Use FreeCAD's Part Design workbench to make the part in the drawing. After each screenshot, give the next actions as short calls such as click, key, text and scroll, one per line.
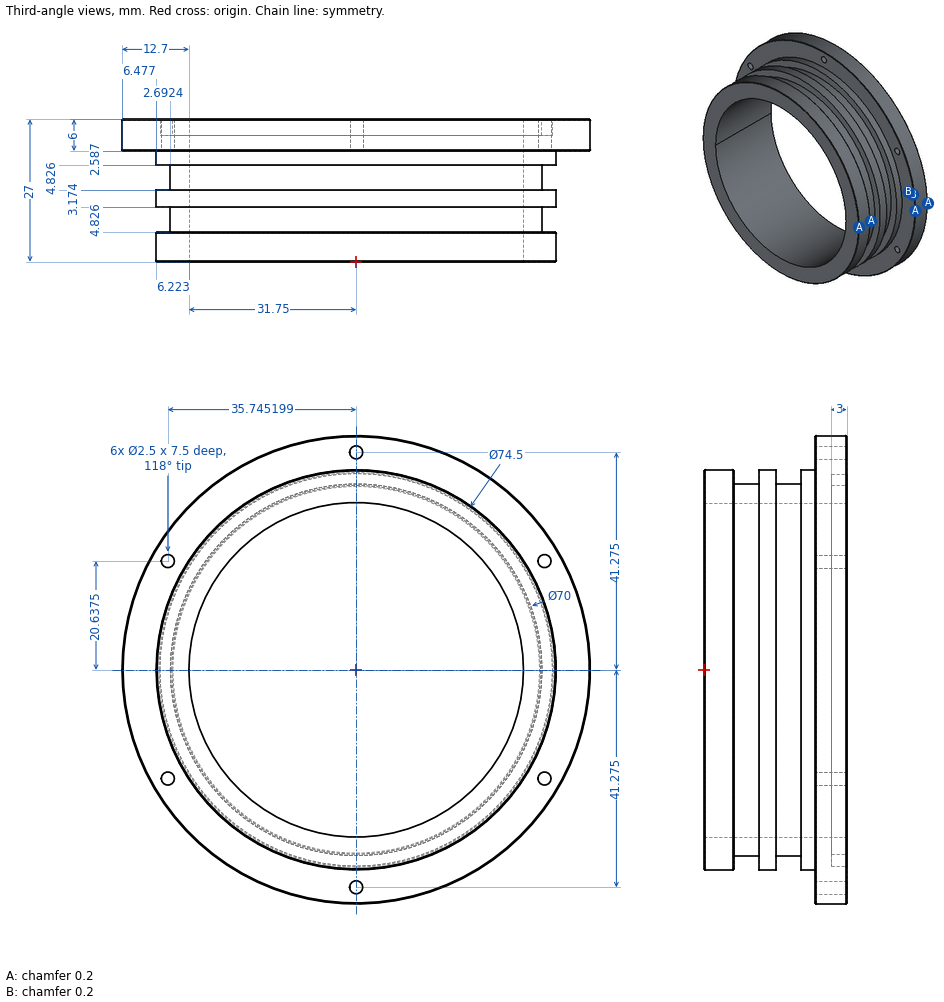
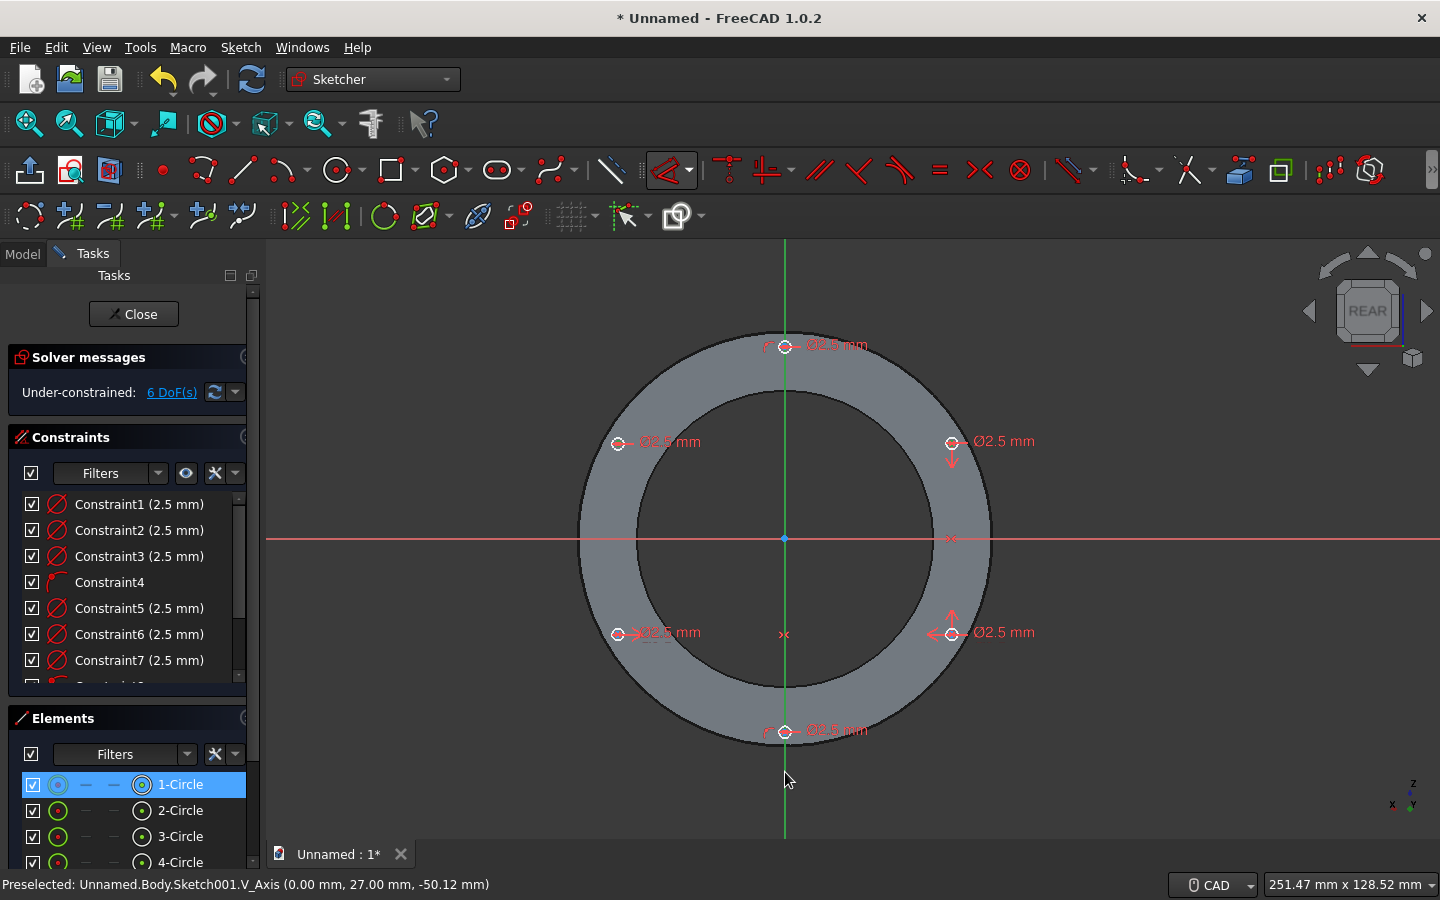
click(980, 170)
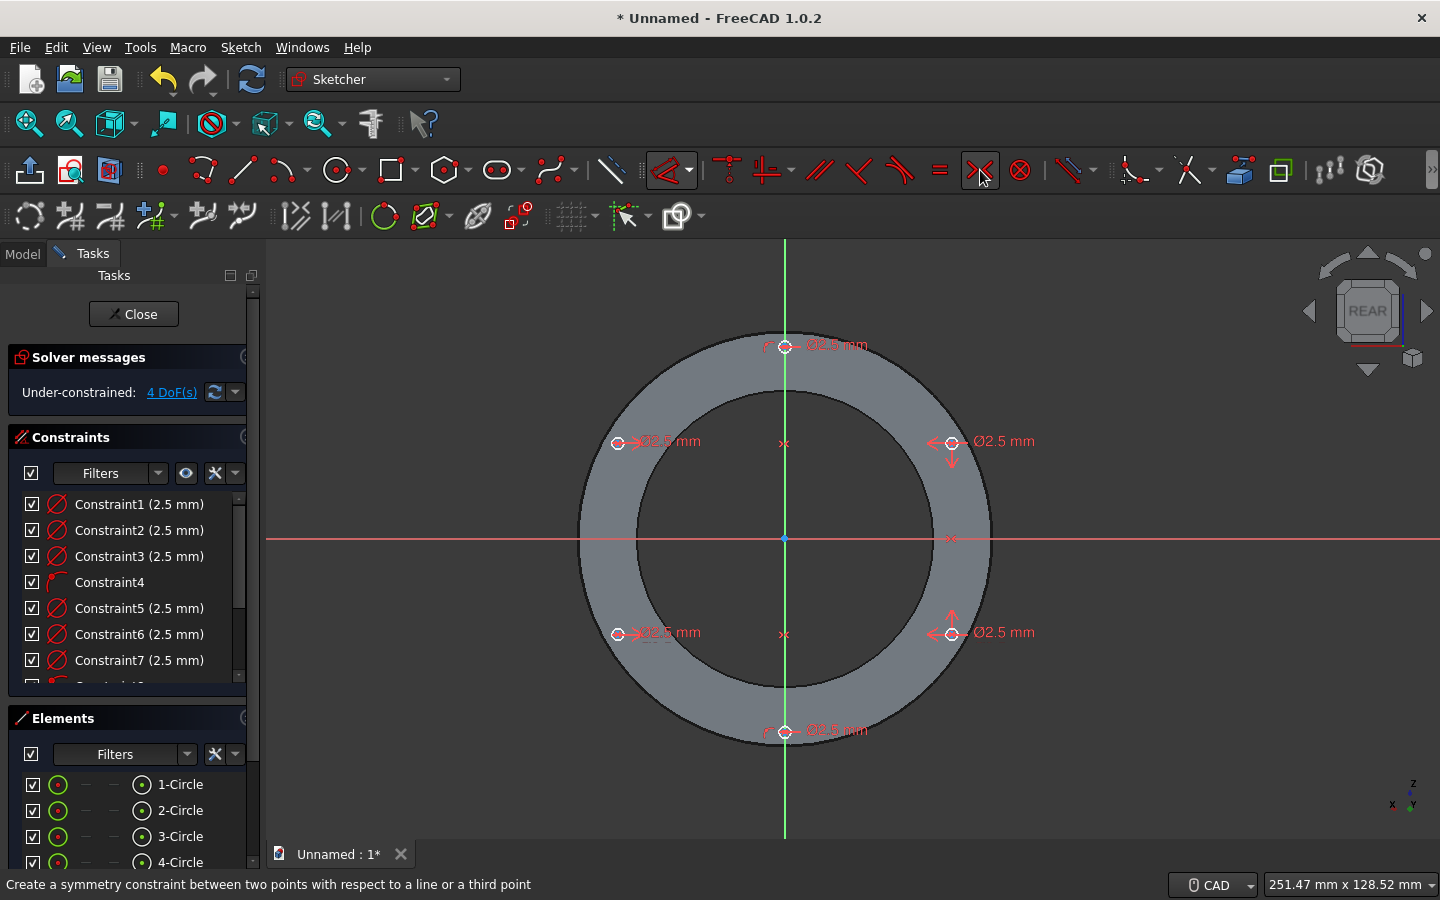
click(785, 732)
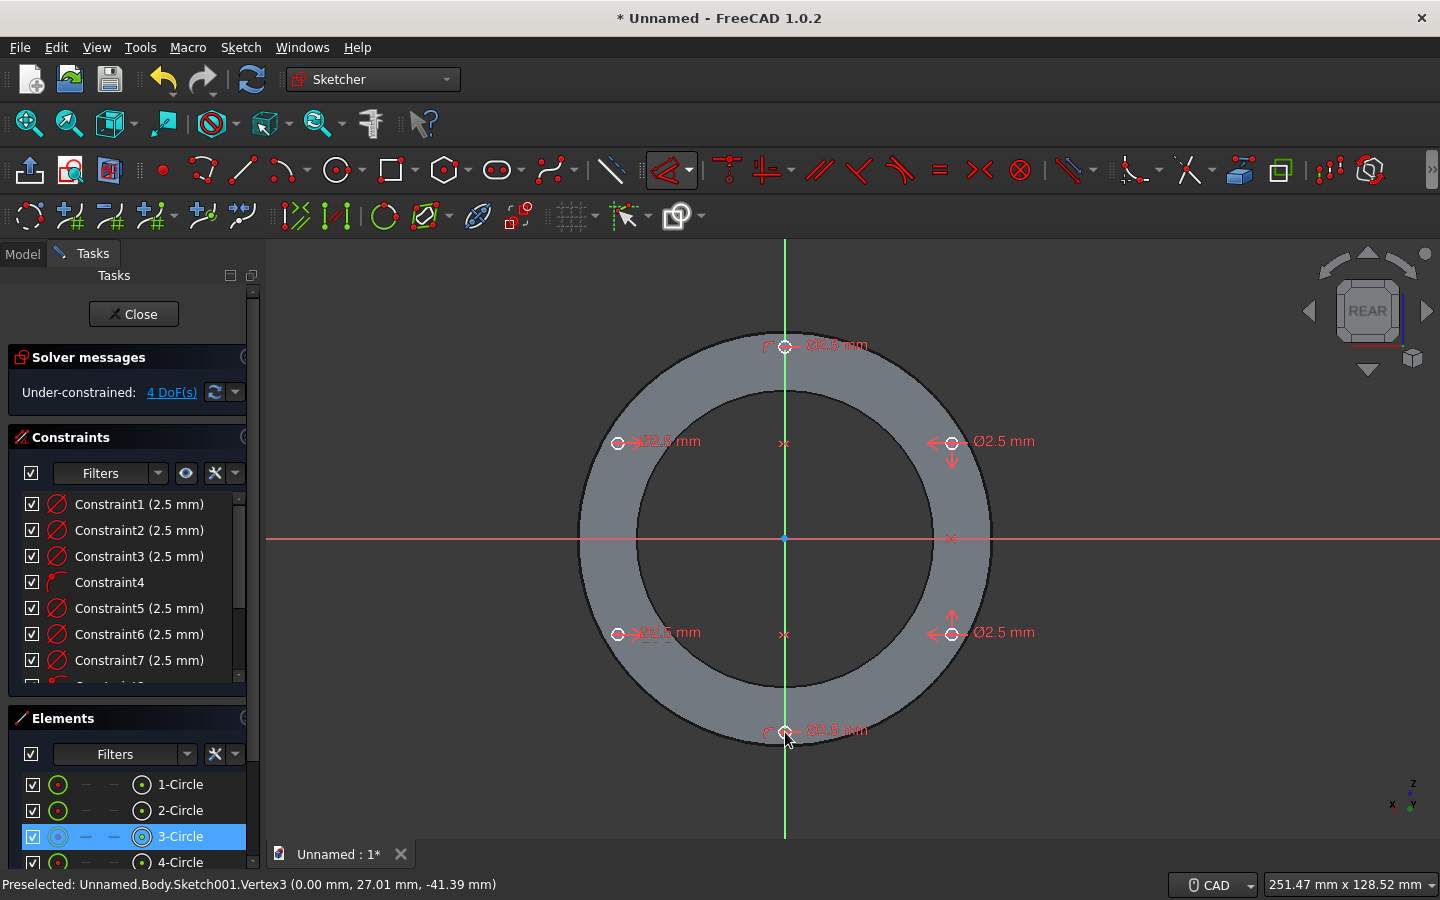
key(i)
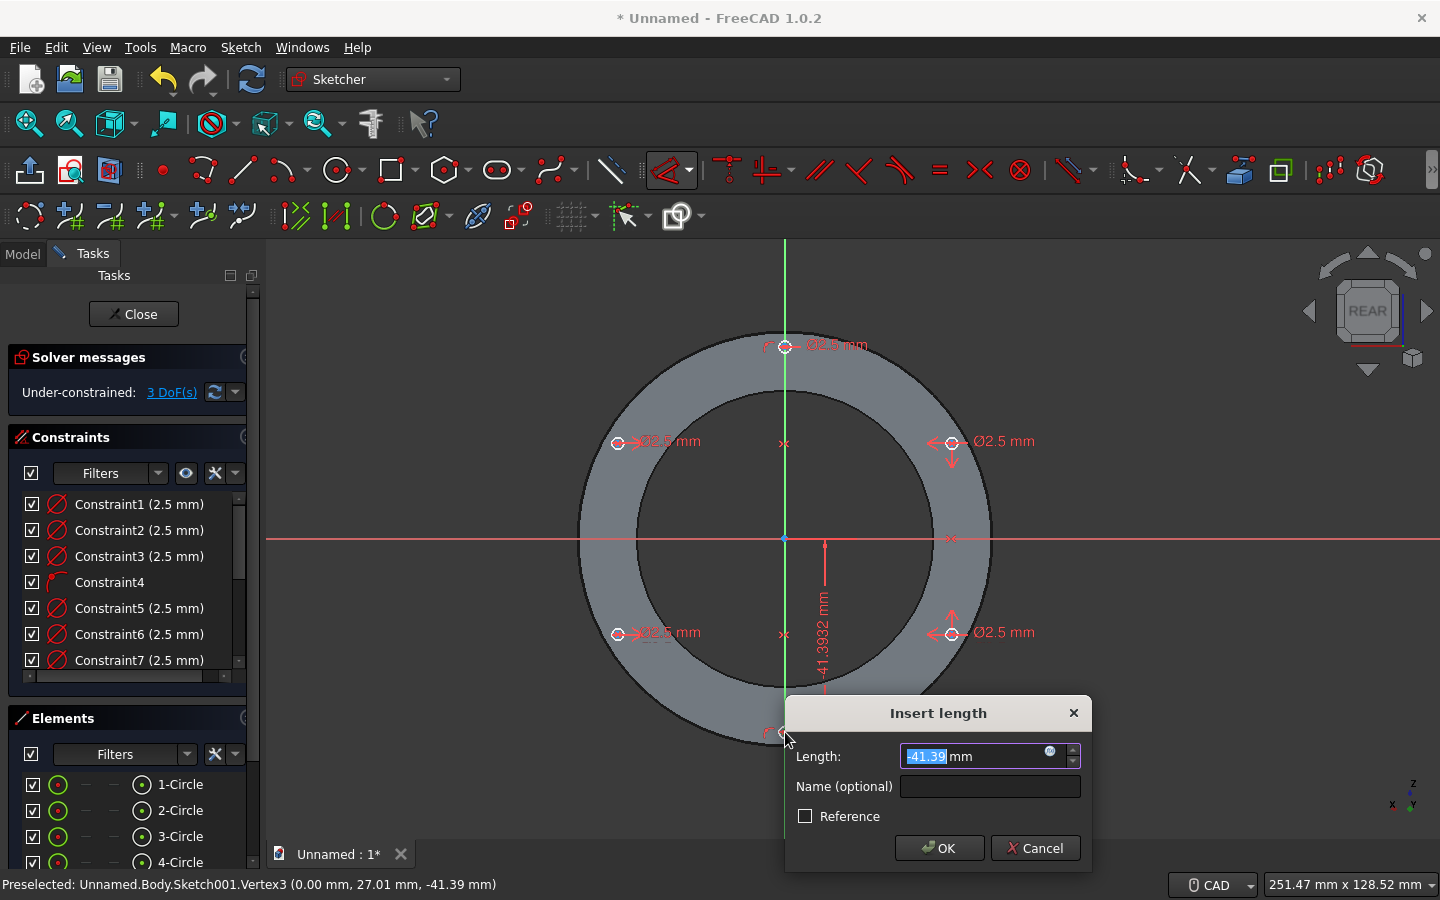
text(-41.275)
key(Return)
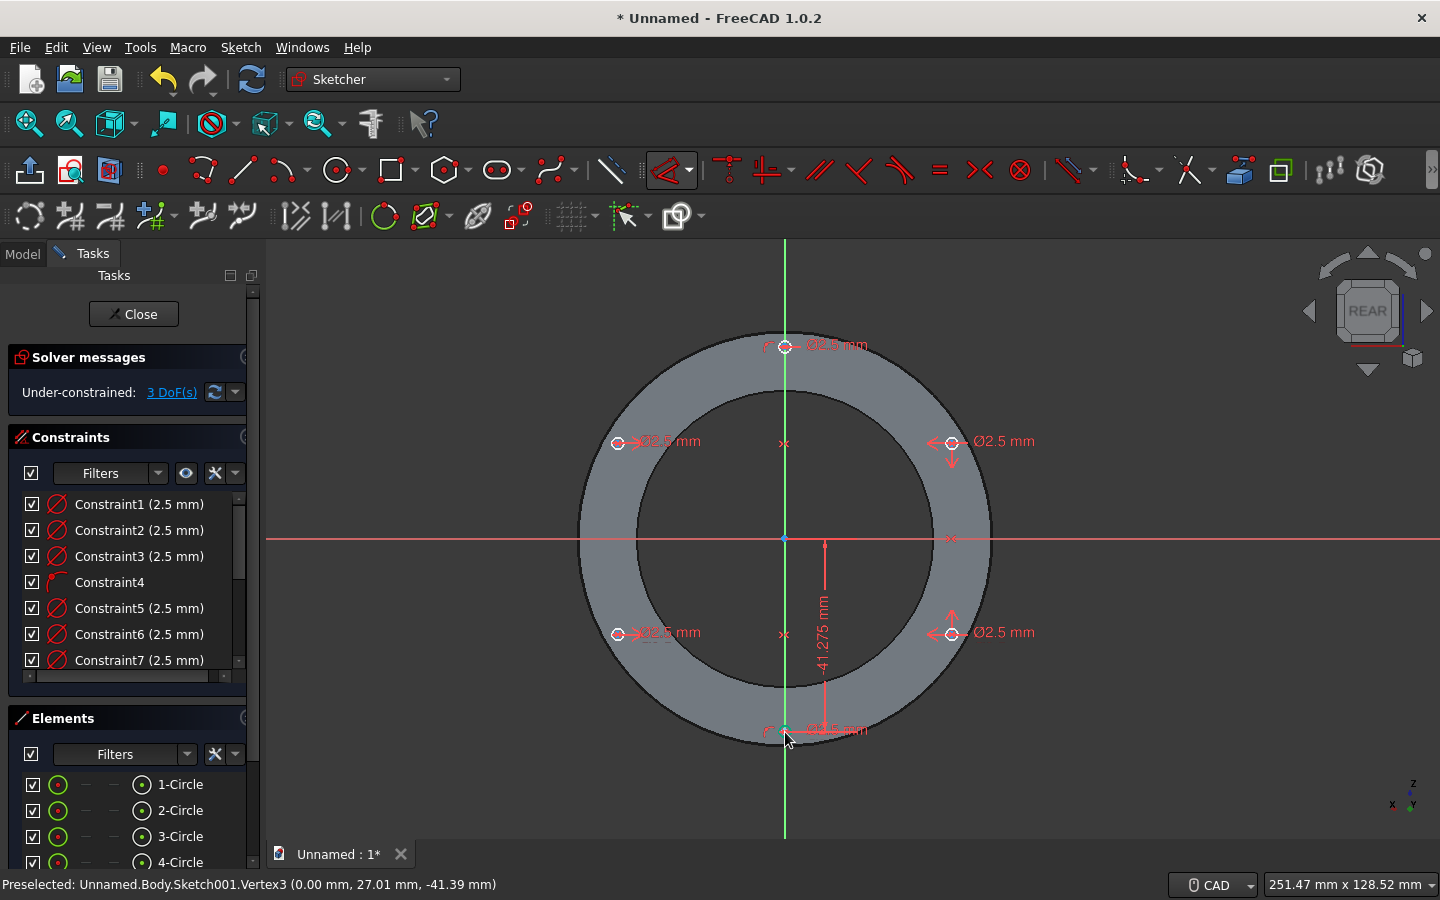
click(785, 347)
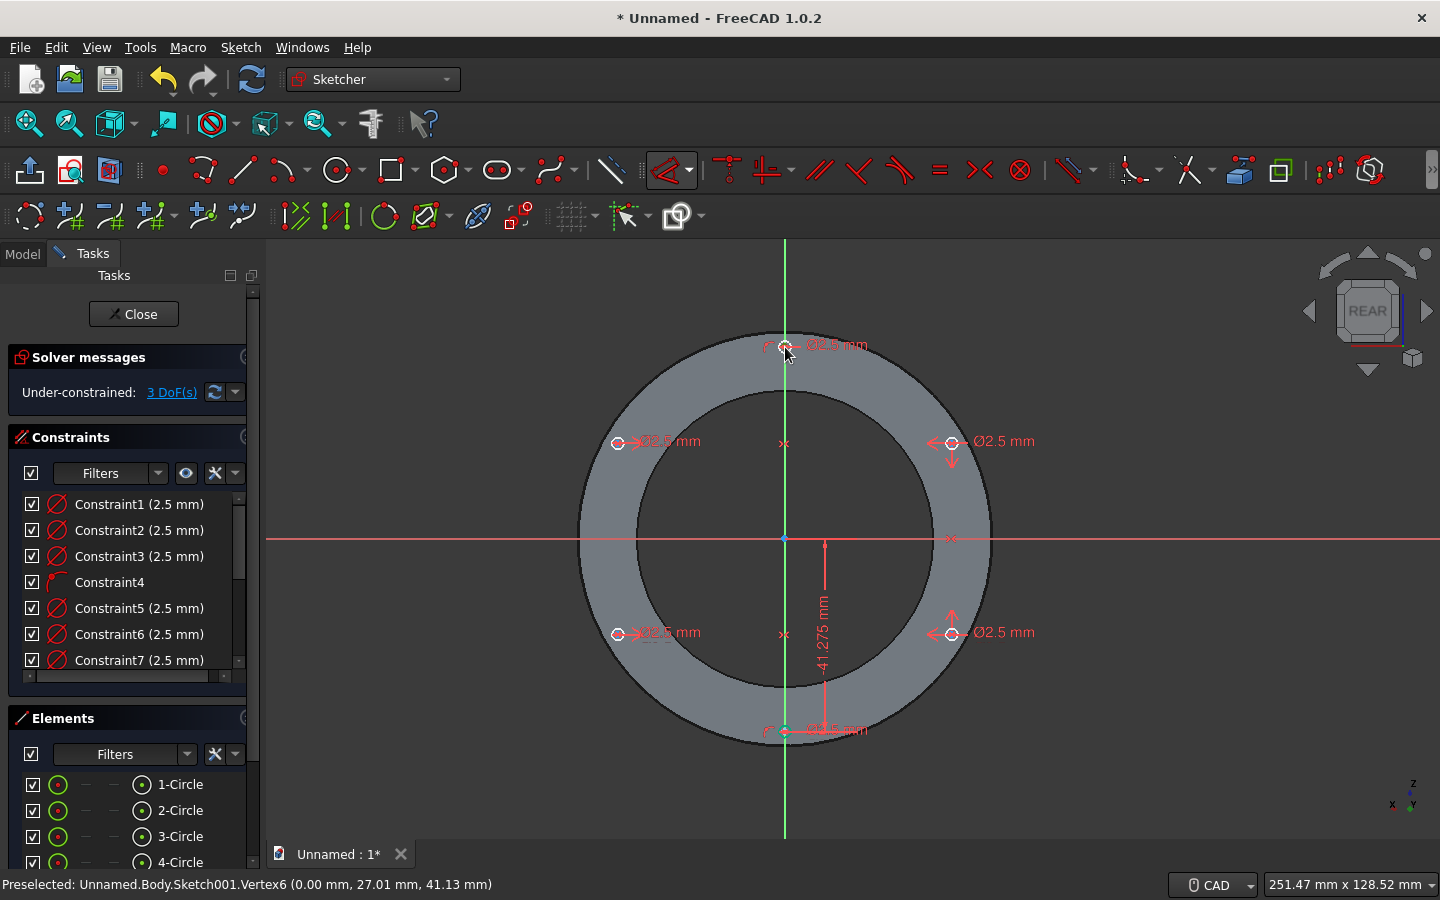
click(692, 170)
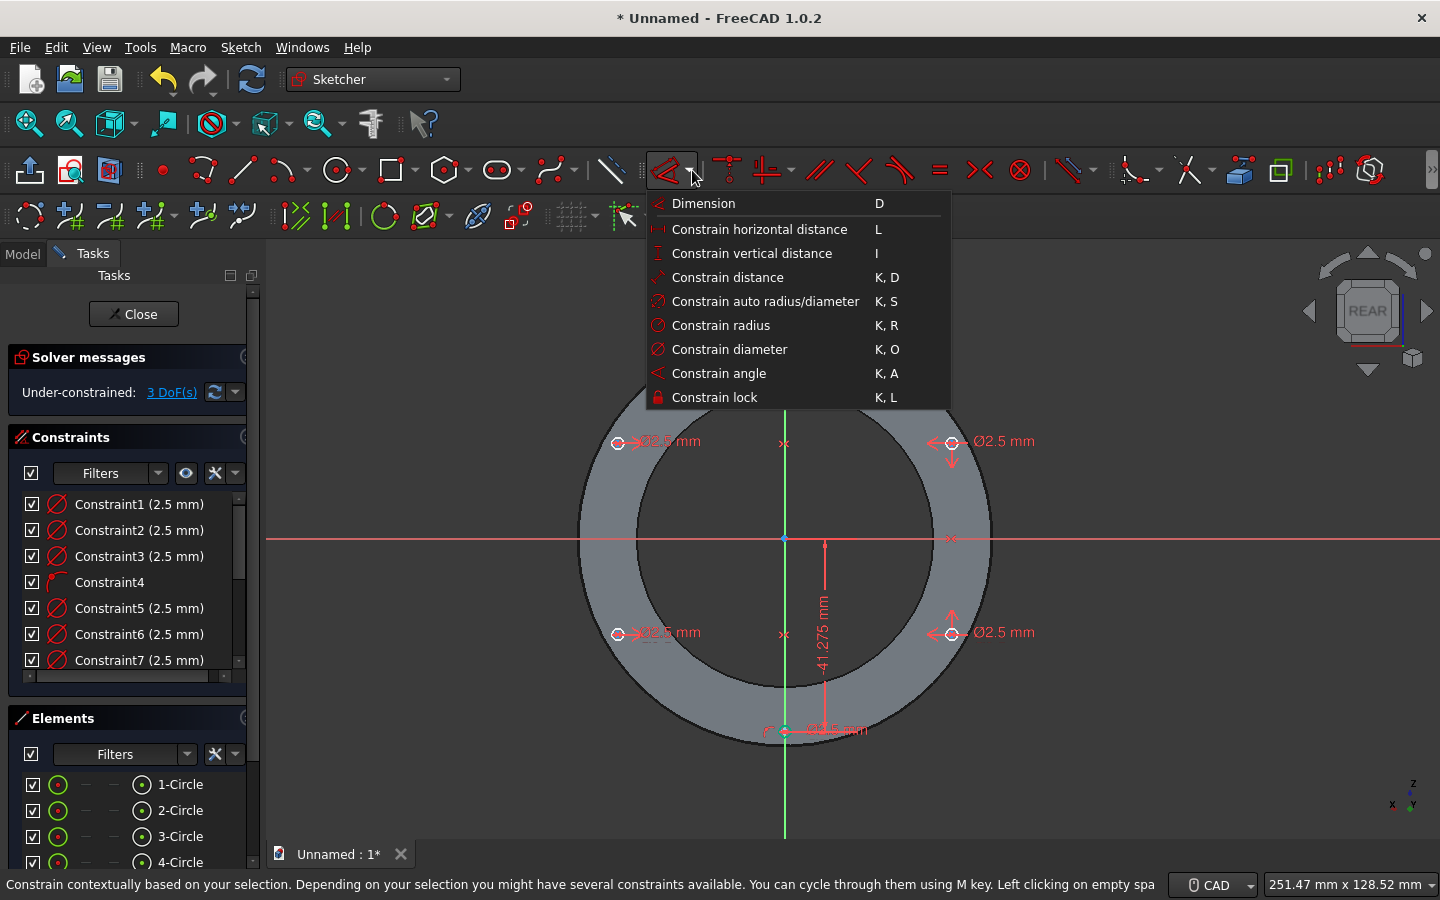
click(799, 253)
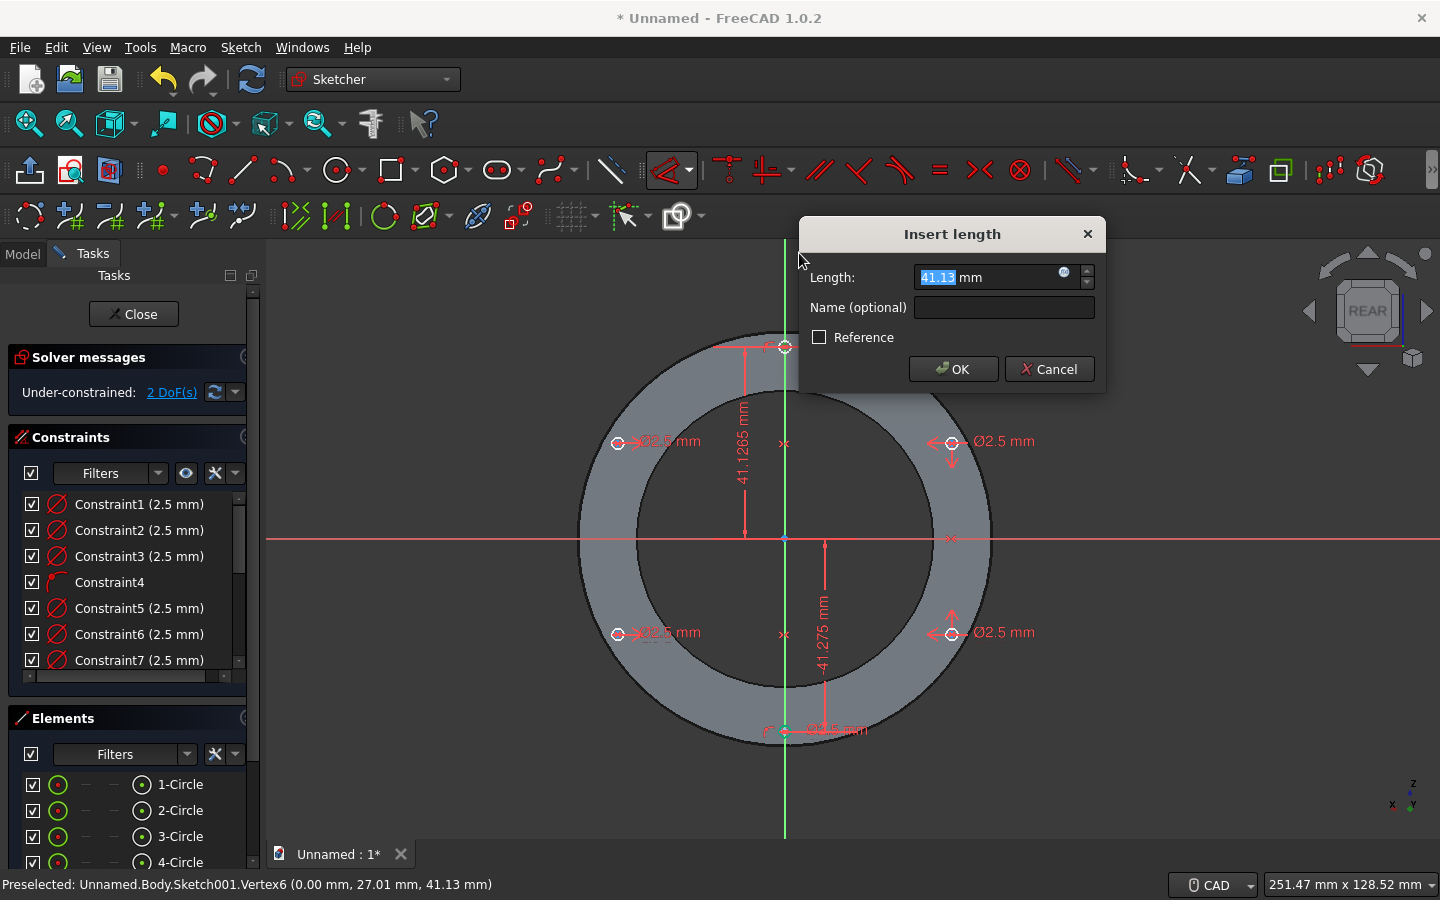
text(41.275)
key(Return)